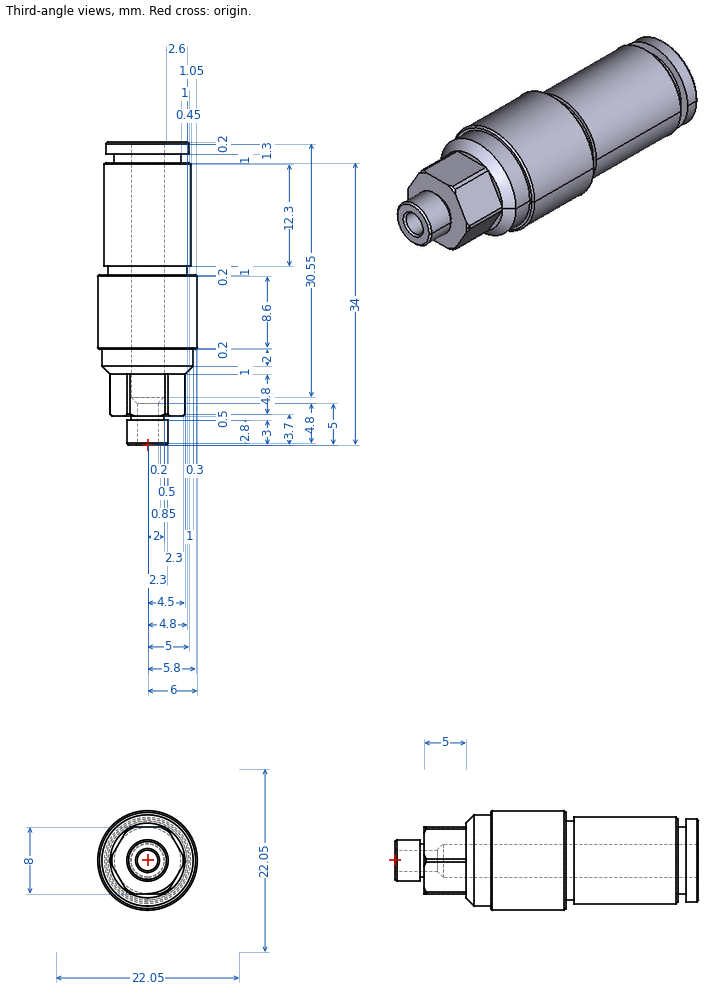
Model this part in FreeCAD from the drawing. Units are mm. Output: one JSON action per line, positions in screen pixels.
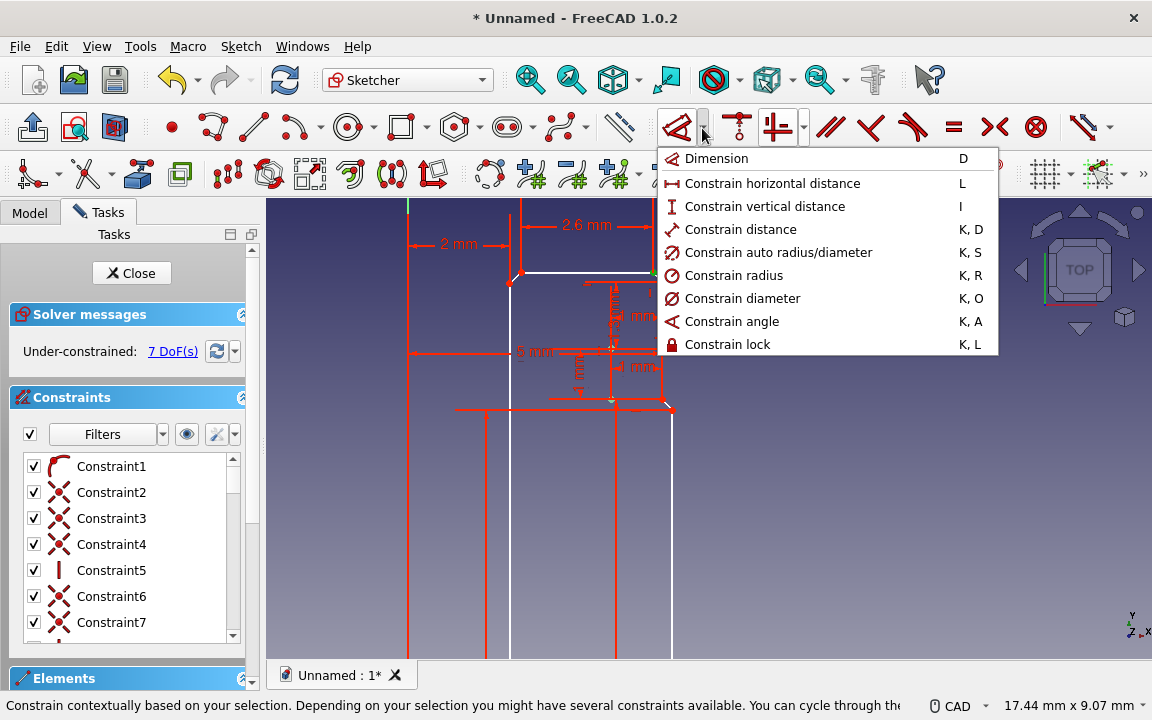
{"action": "left_click", "coordinate": [828, 184]}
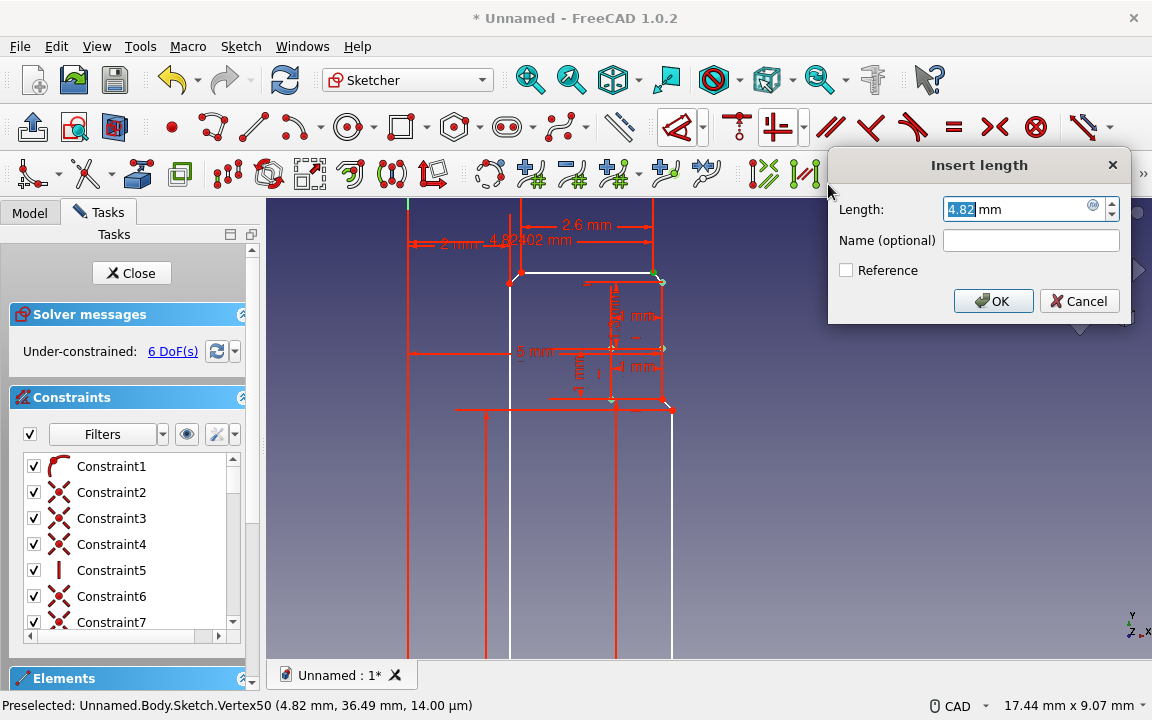
{"action": "type", "text": "4.8"}
{"action": "key", "text": "Return"}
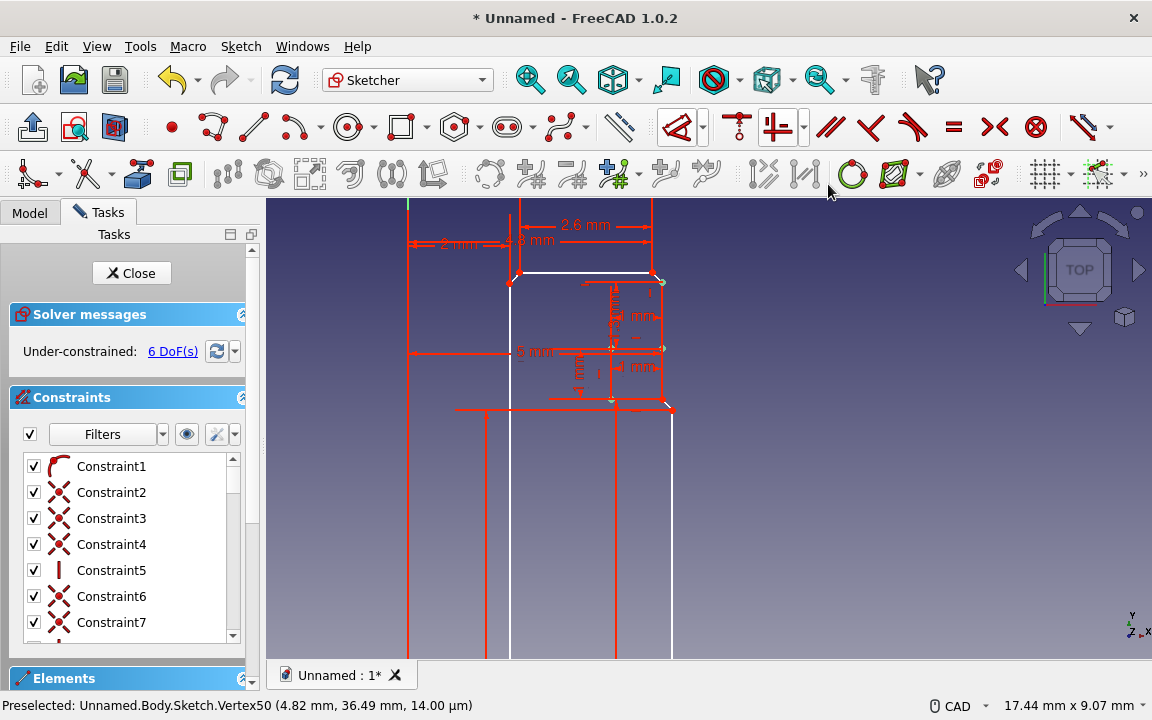
{"action": "scroll", "coordinate": [656, 276], "scroll_direction": "down", "scroll_amount": 9}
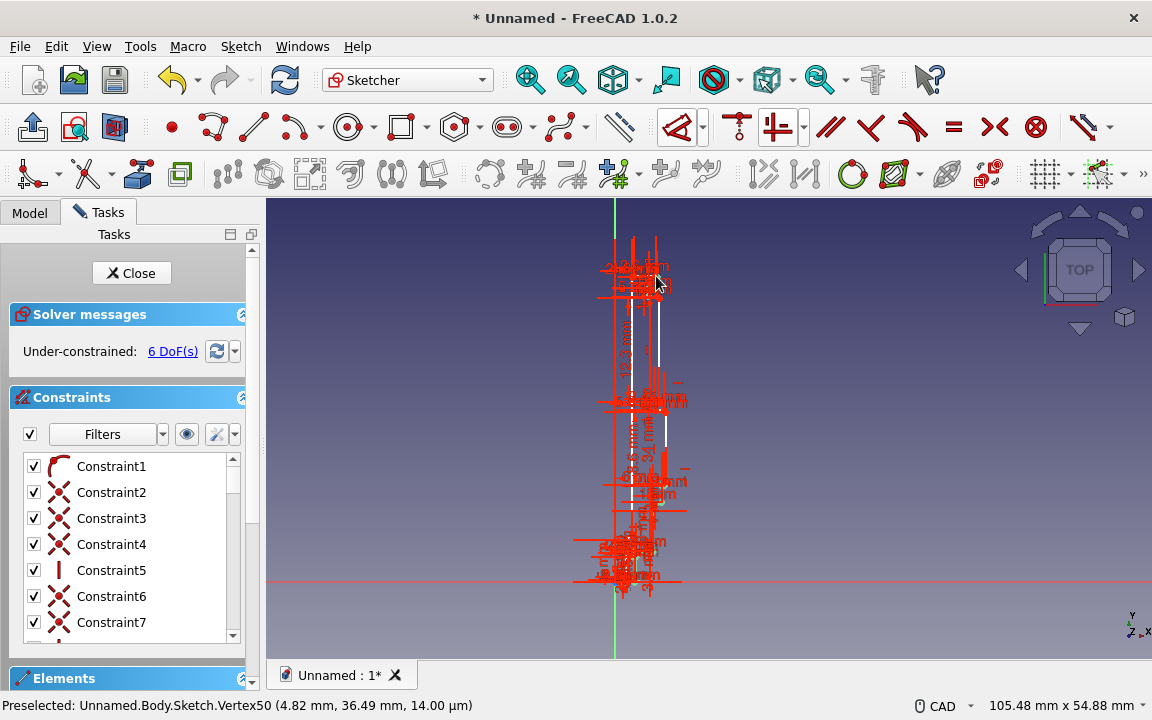
{"action": "scroll", "coordinate": [626, 581], "scroll_direction": "up", "scroll_amount": 16}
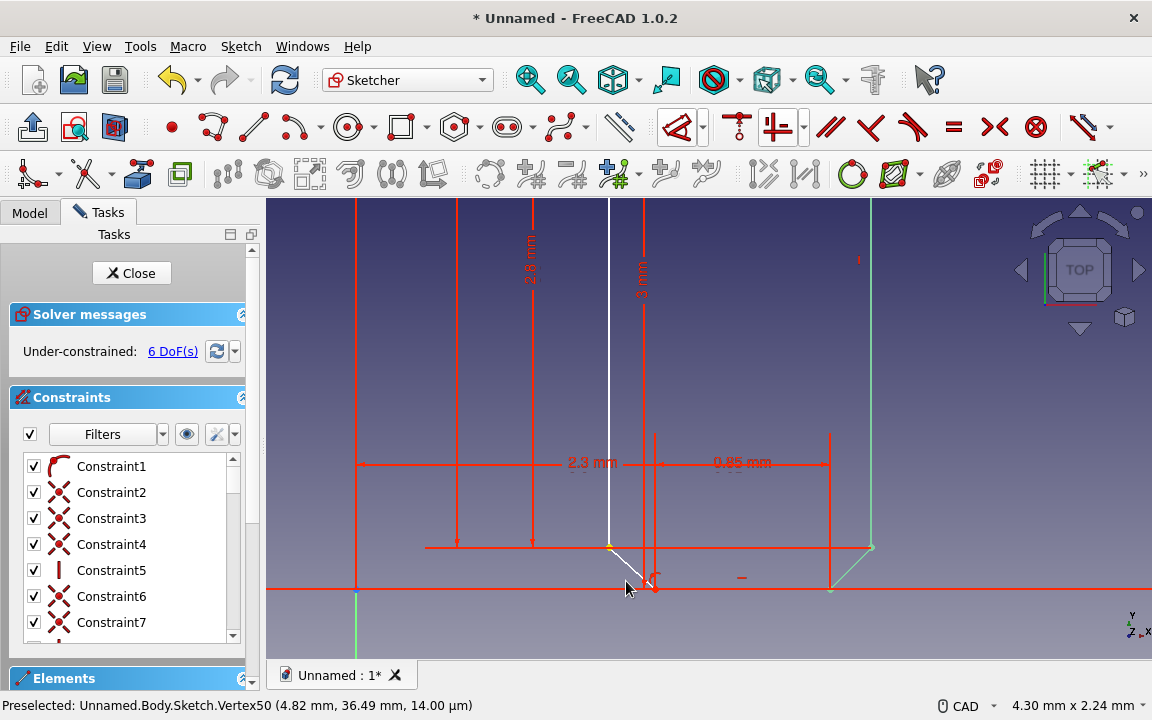
{"action": "left_click", "coordinate": [628, 564]}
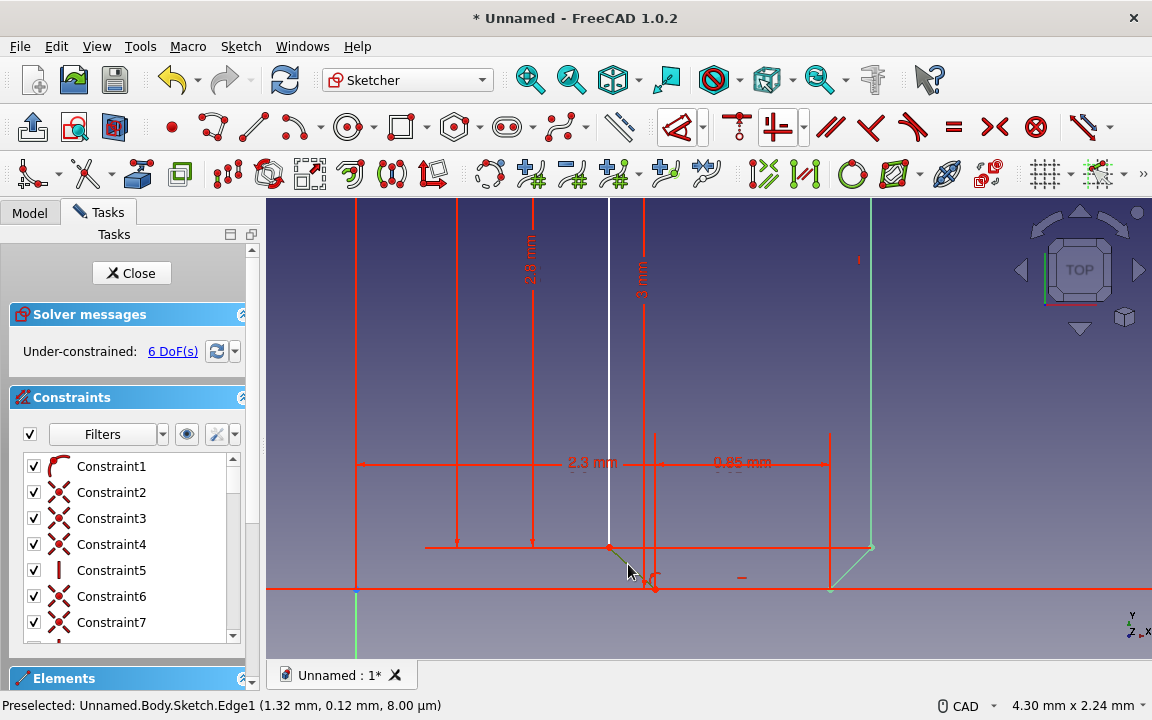
{"action": "left_click", "coordinate": [702, 128]}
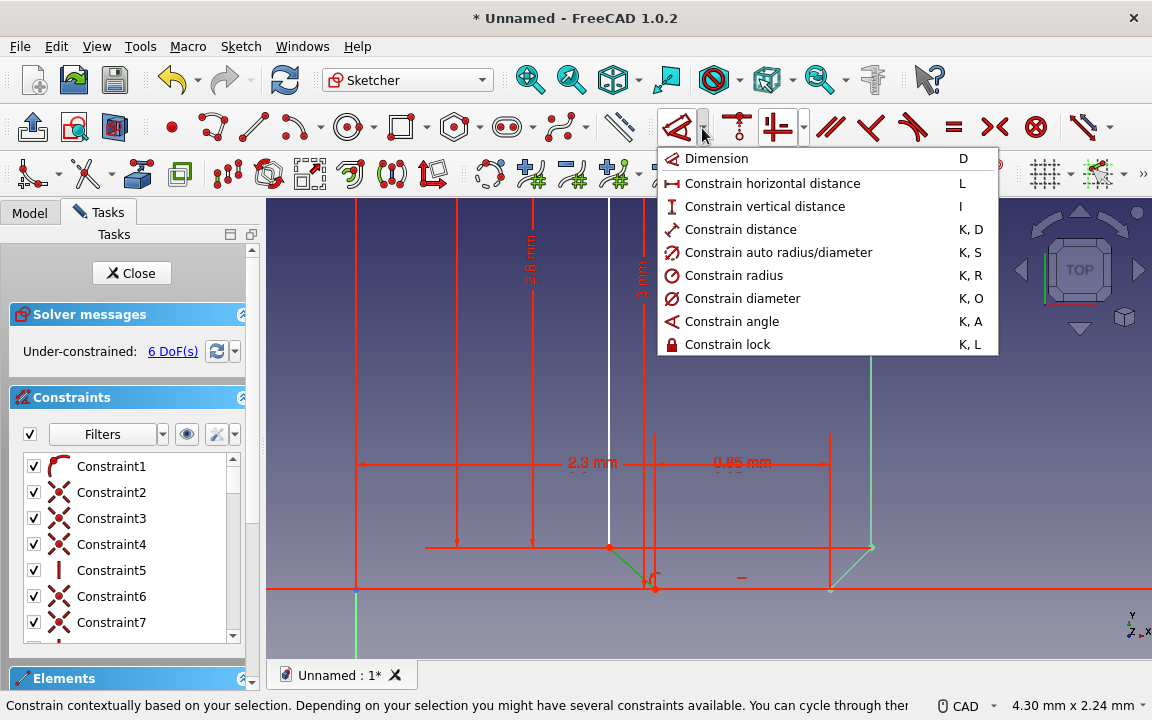
{"action": "left_click", "coordinate": [828, 184]}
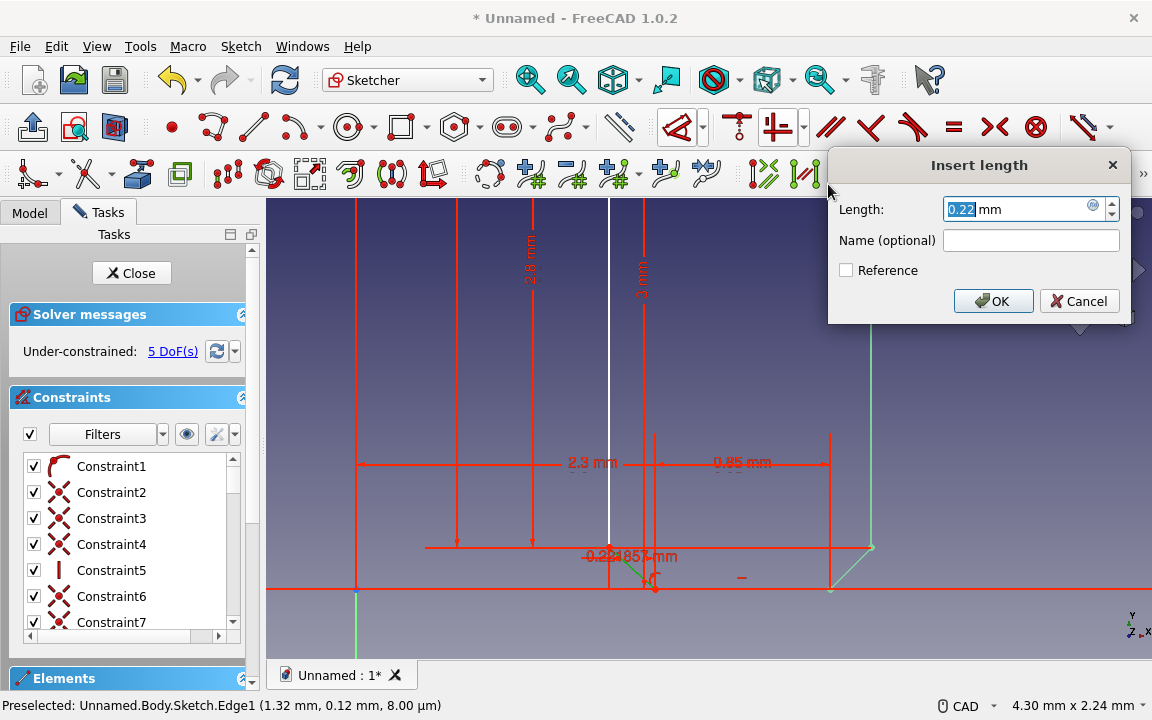
{"action": "type", "text": "0.2"}
{"action": "key", "text": "Return"}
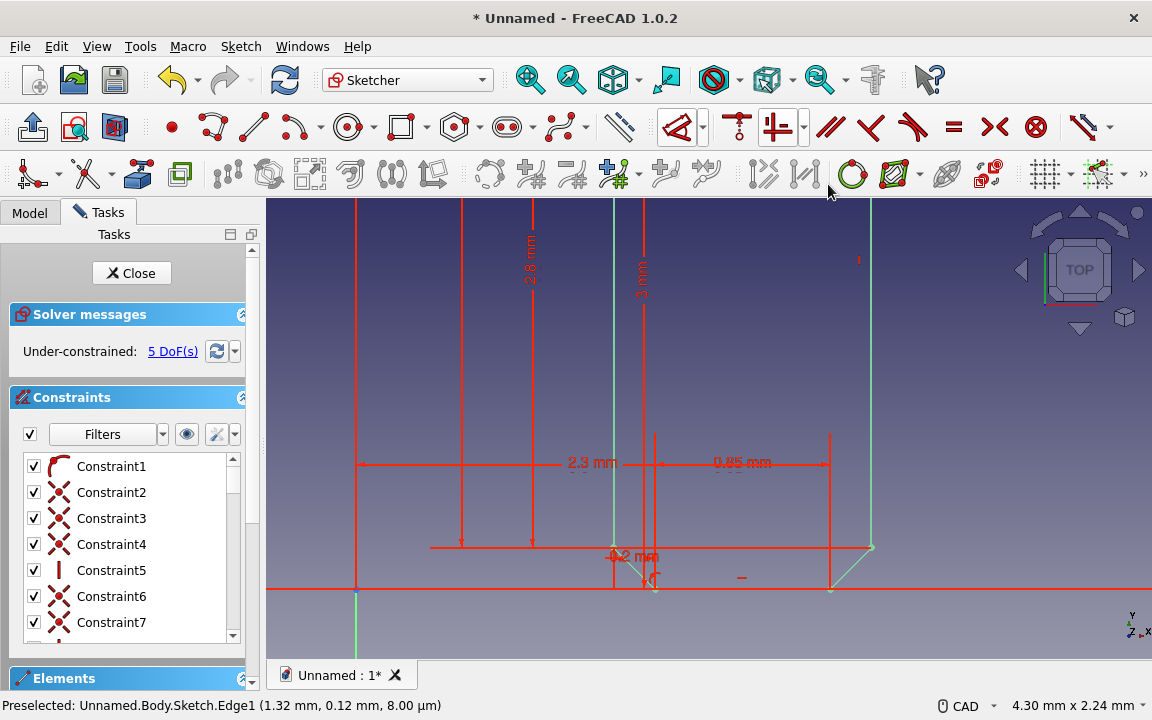
{"action": "scroll", "coordinate": [626, 581], "scroll_direction": "down", "scroll_amount": 16}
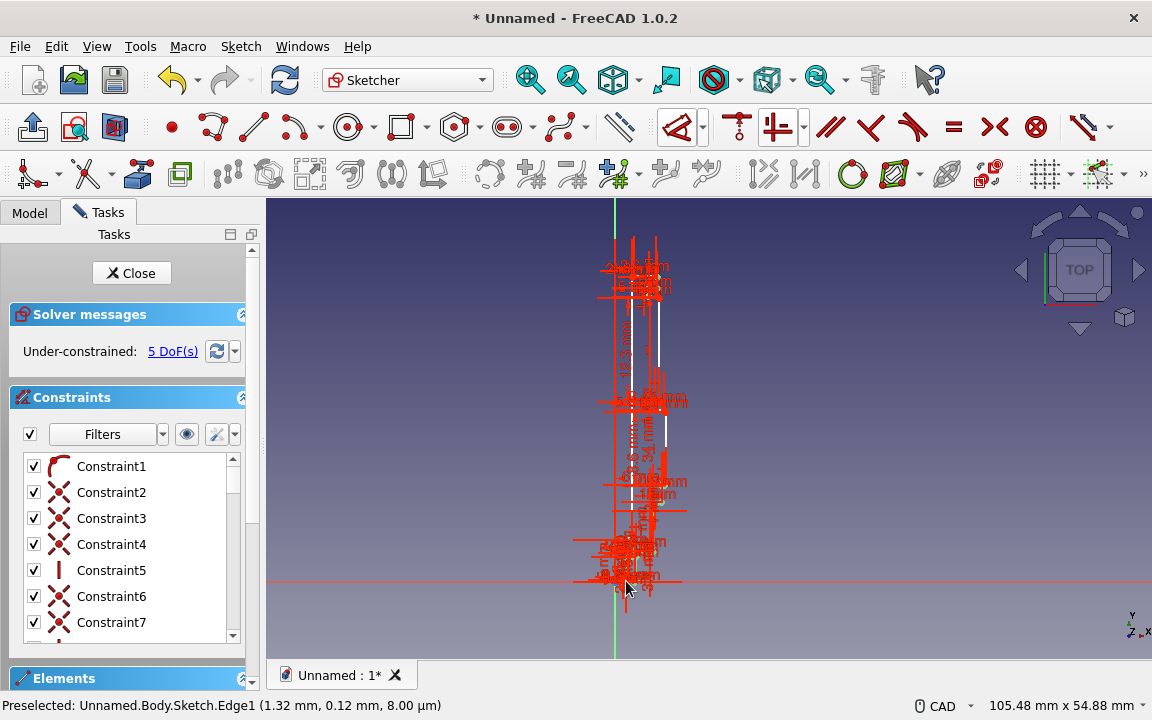
{"action": "scroll", "coordinate": [665, 485], "scroll_direction": "up", "scroll_amount": 16}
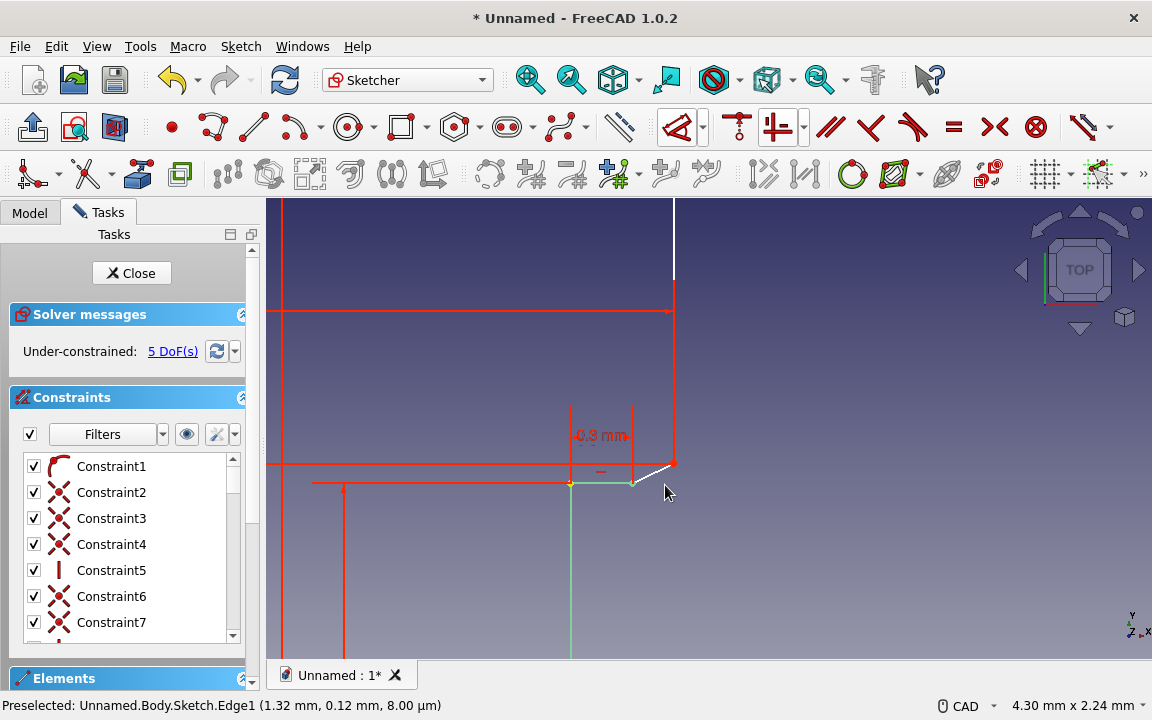
{"action": "left_click", "coordinate": [645, 477]}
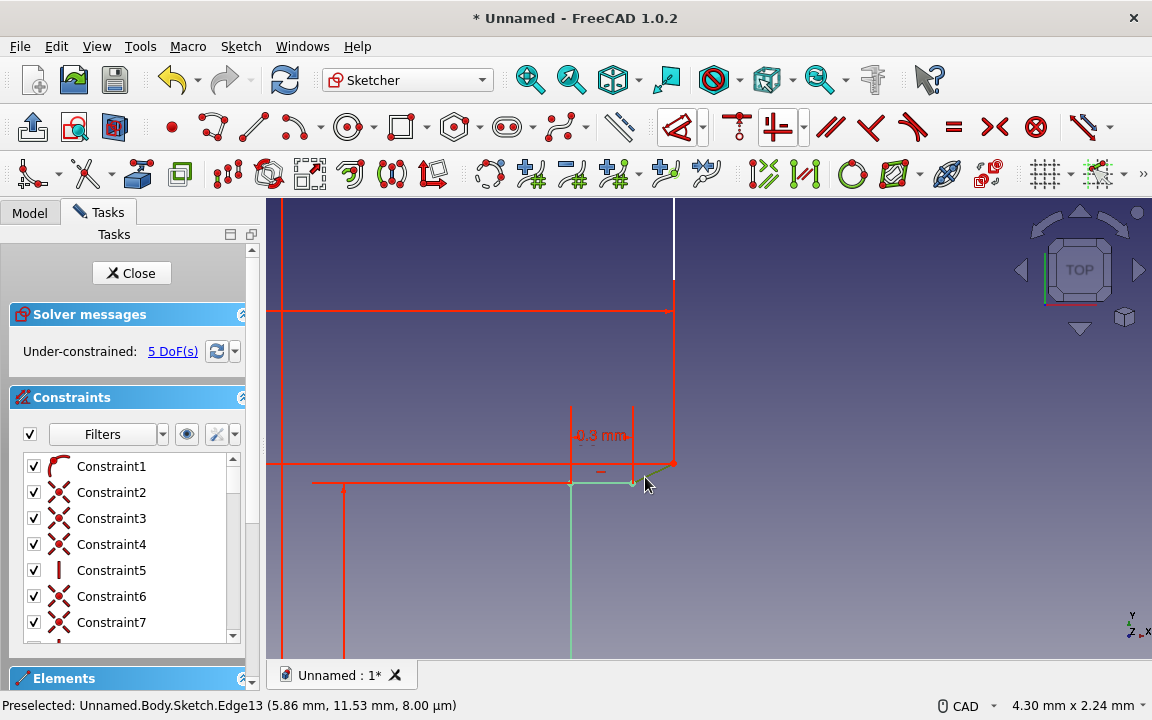
{"action": "left_click", "coordinate": [702, 128]}